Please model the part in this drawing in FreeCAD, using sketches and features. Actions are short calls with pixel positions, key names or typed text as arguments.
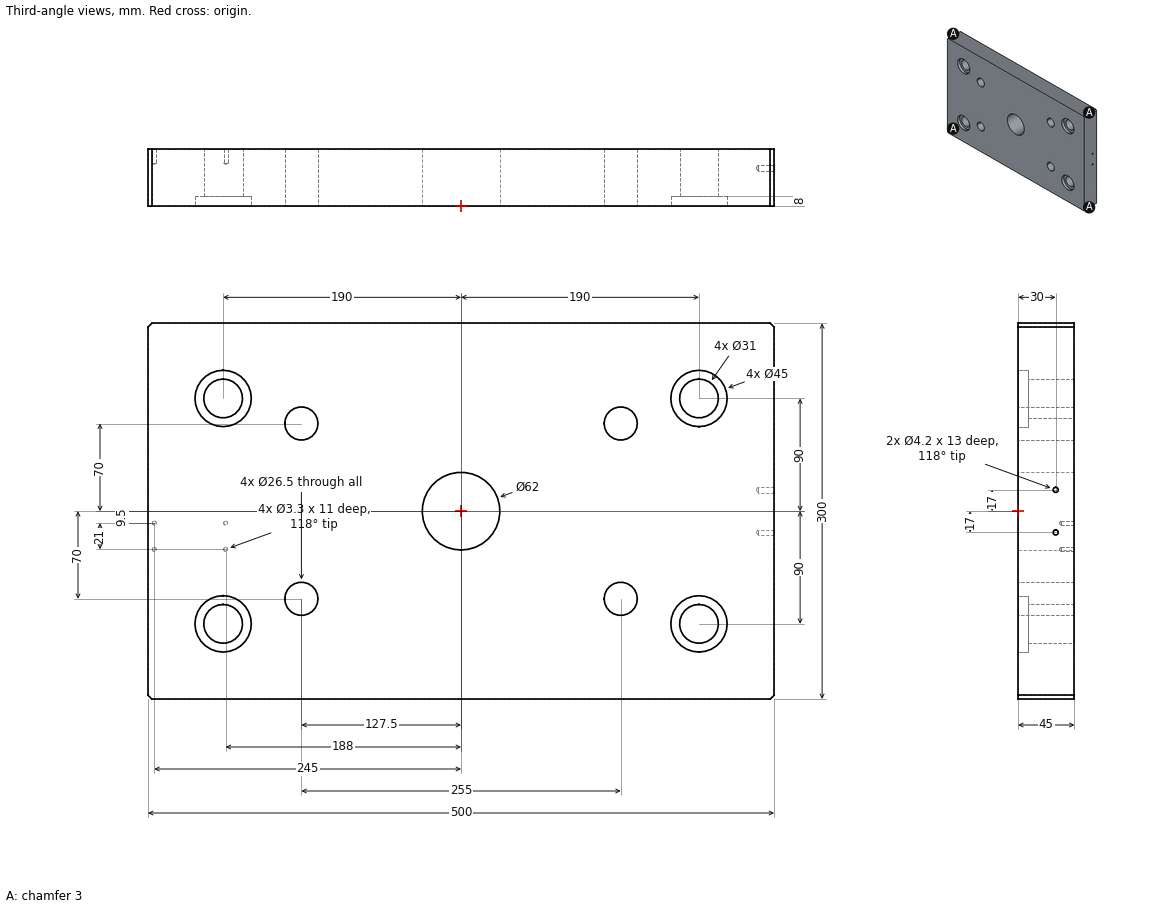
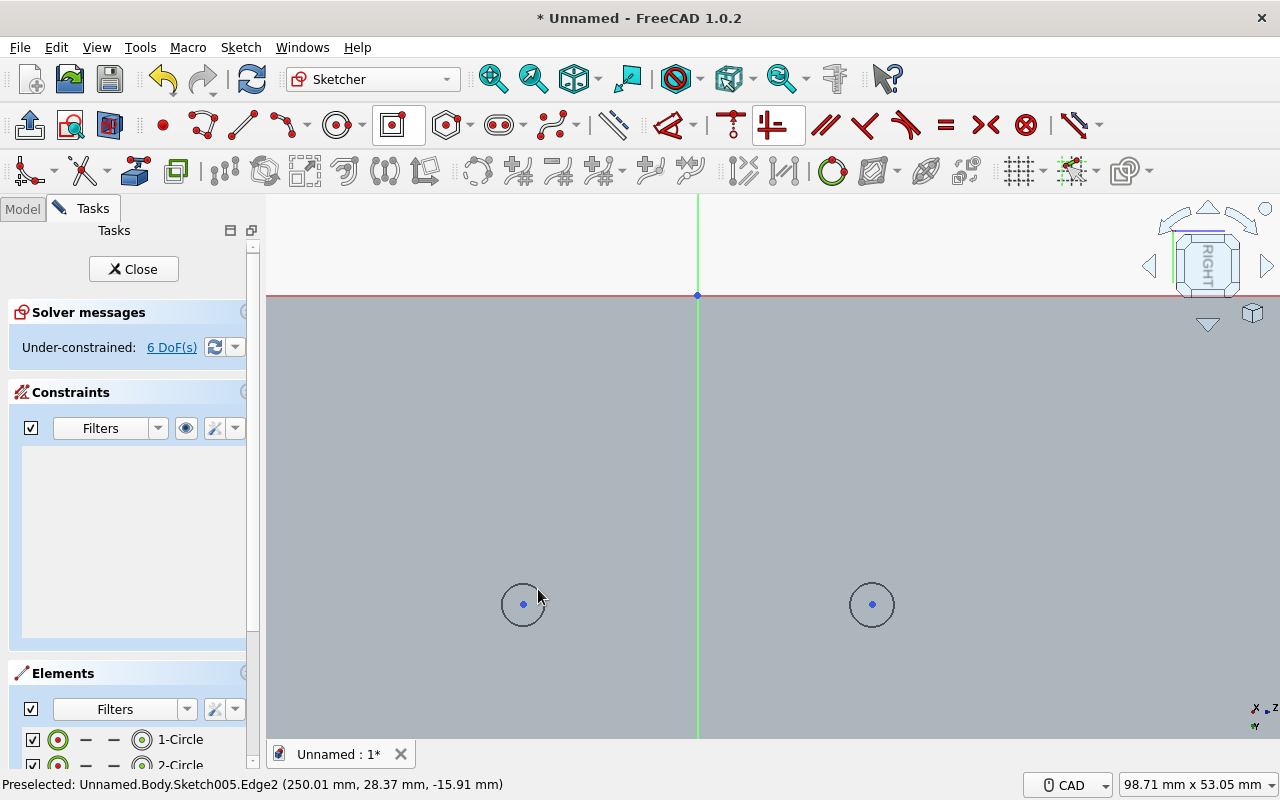
click(887, 589)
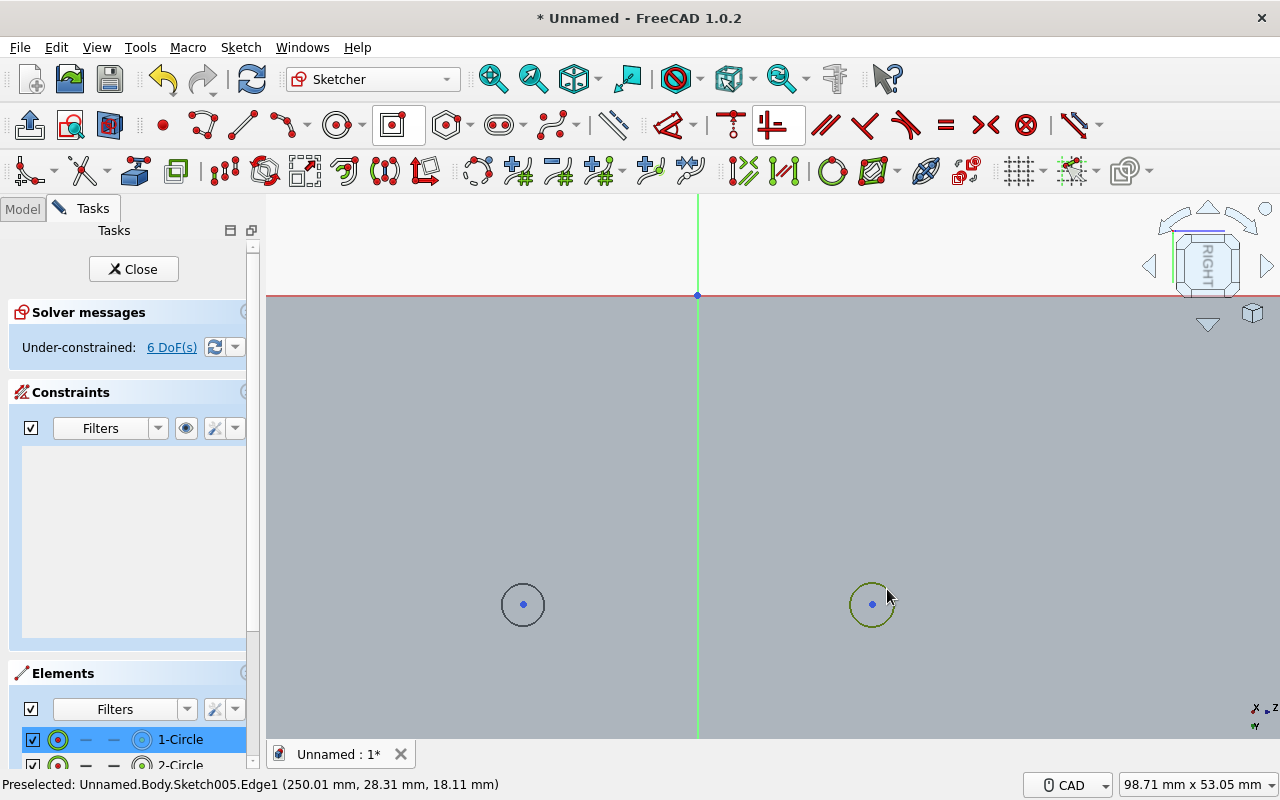
click(538, 590)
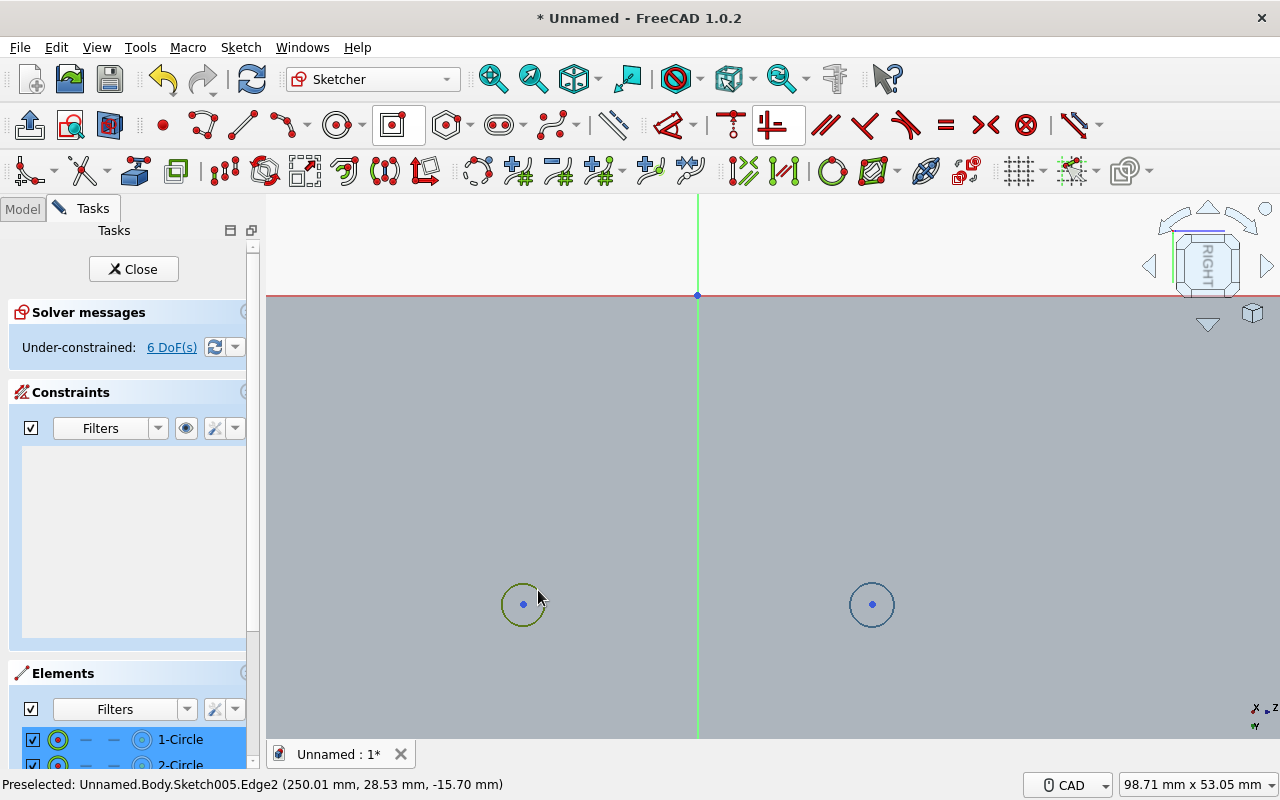
click(946, 126)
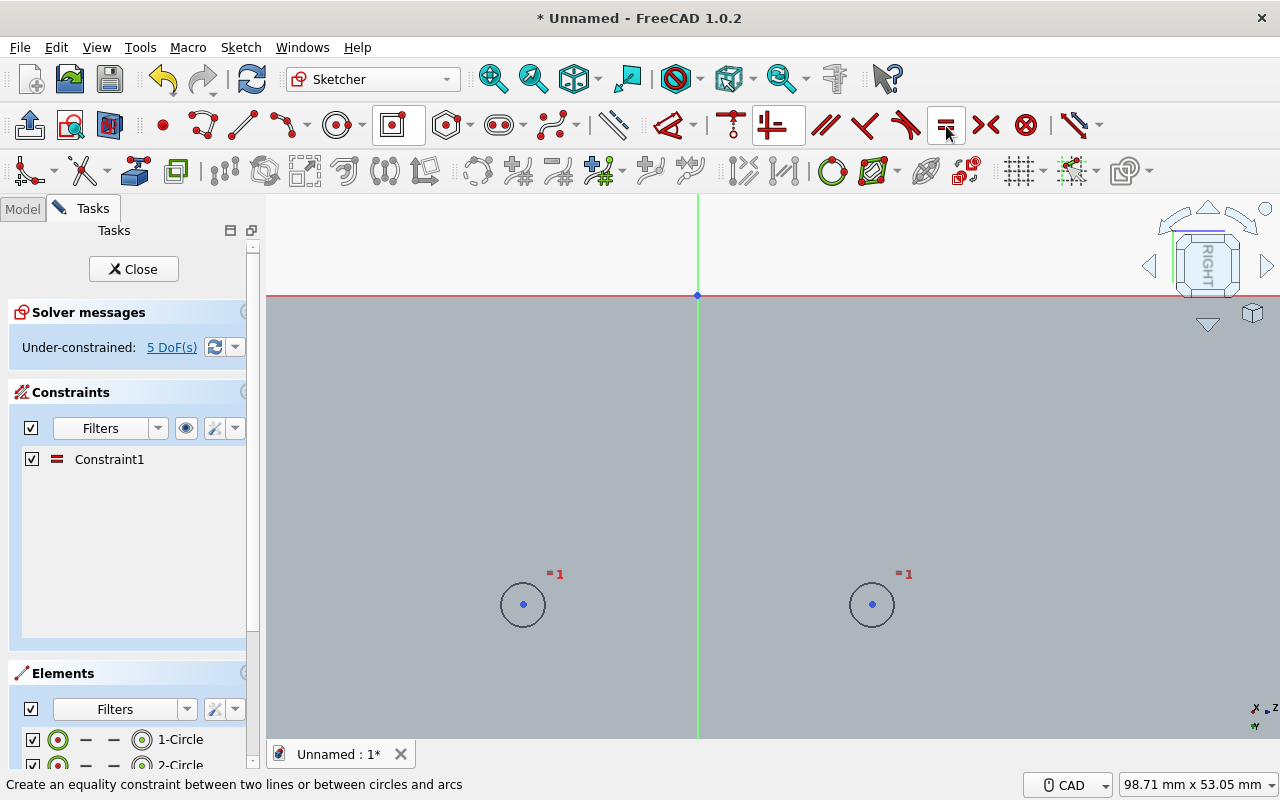
click(872, 605)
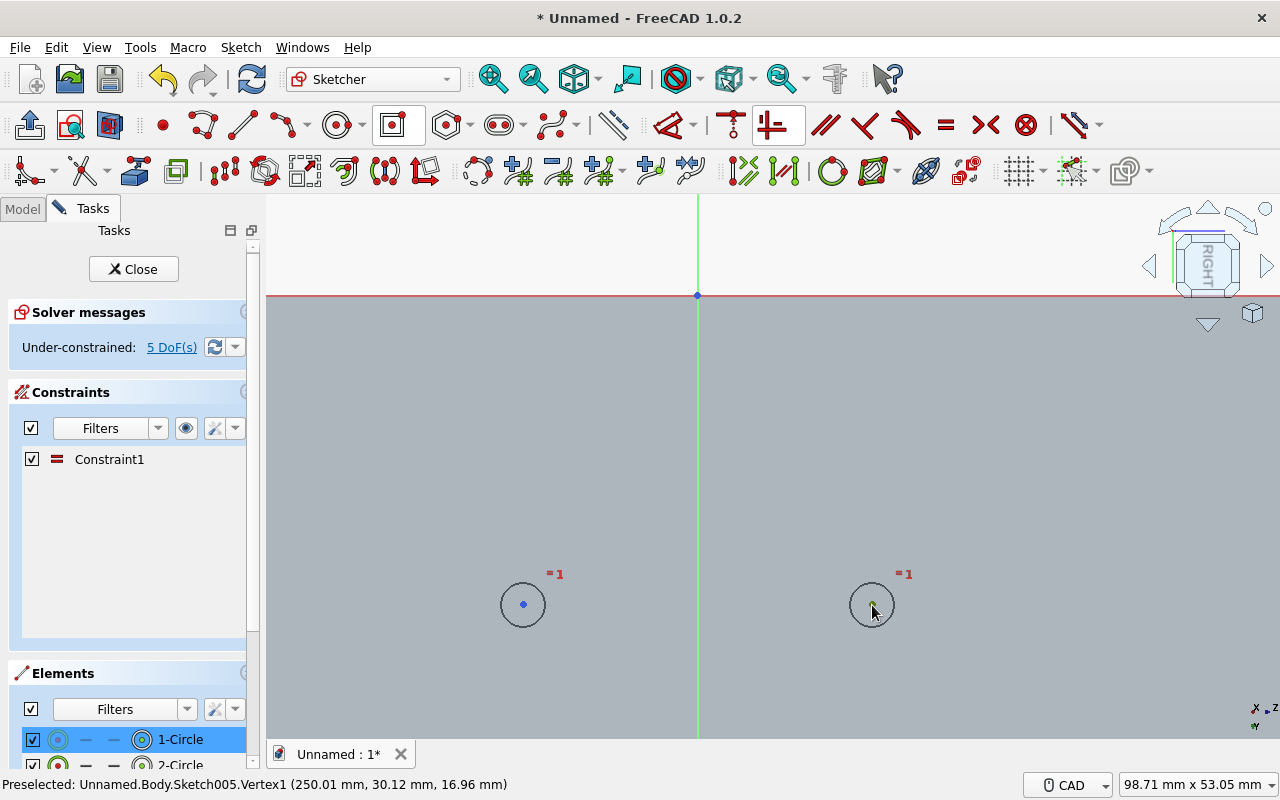
click(523, 605)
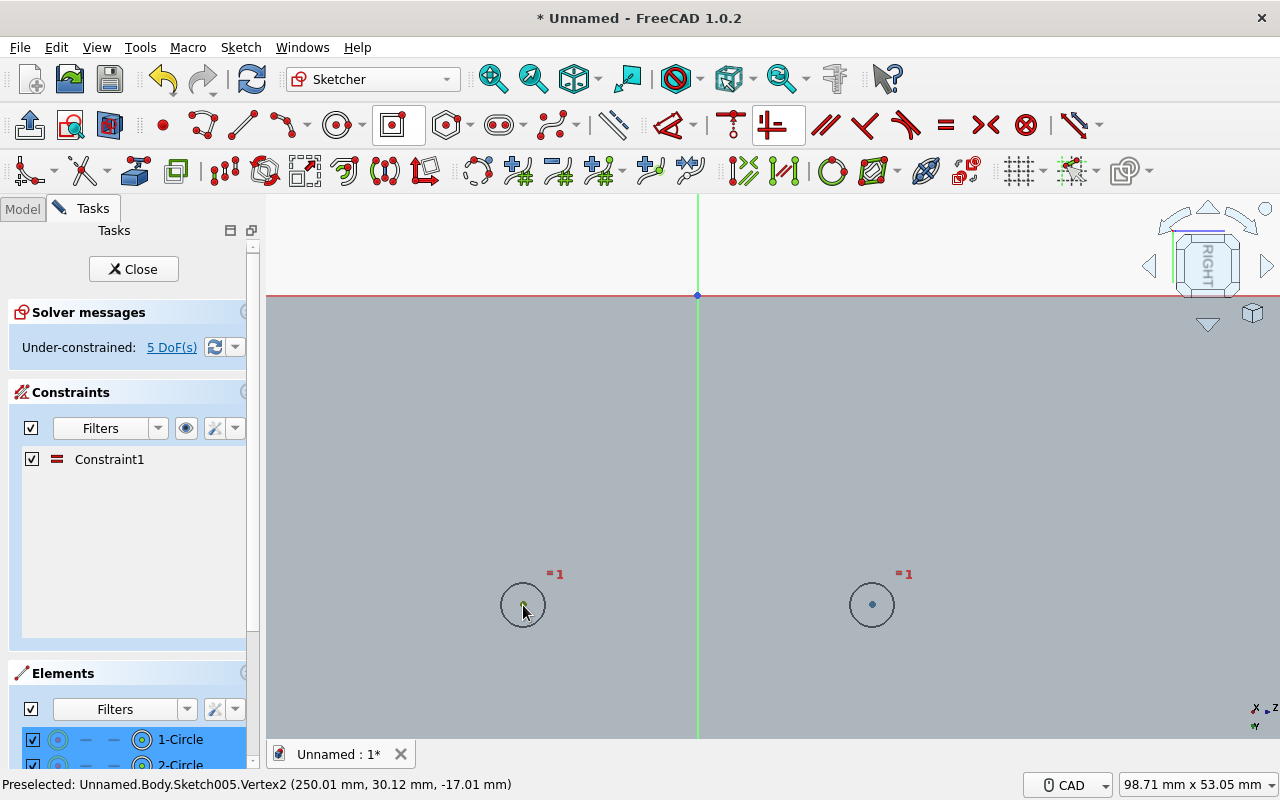
key(h)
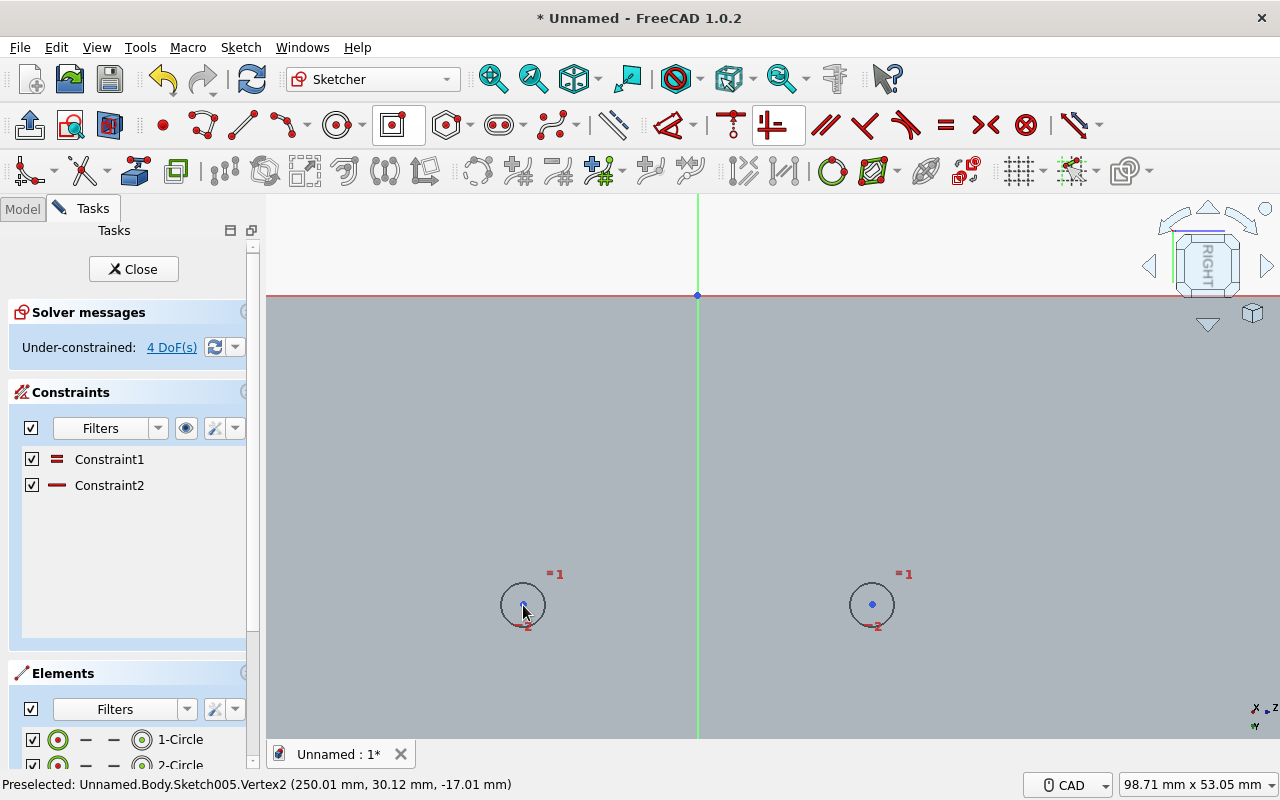
key(d)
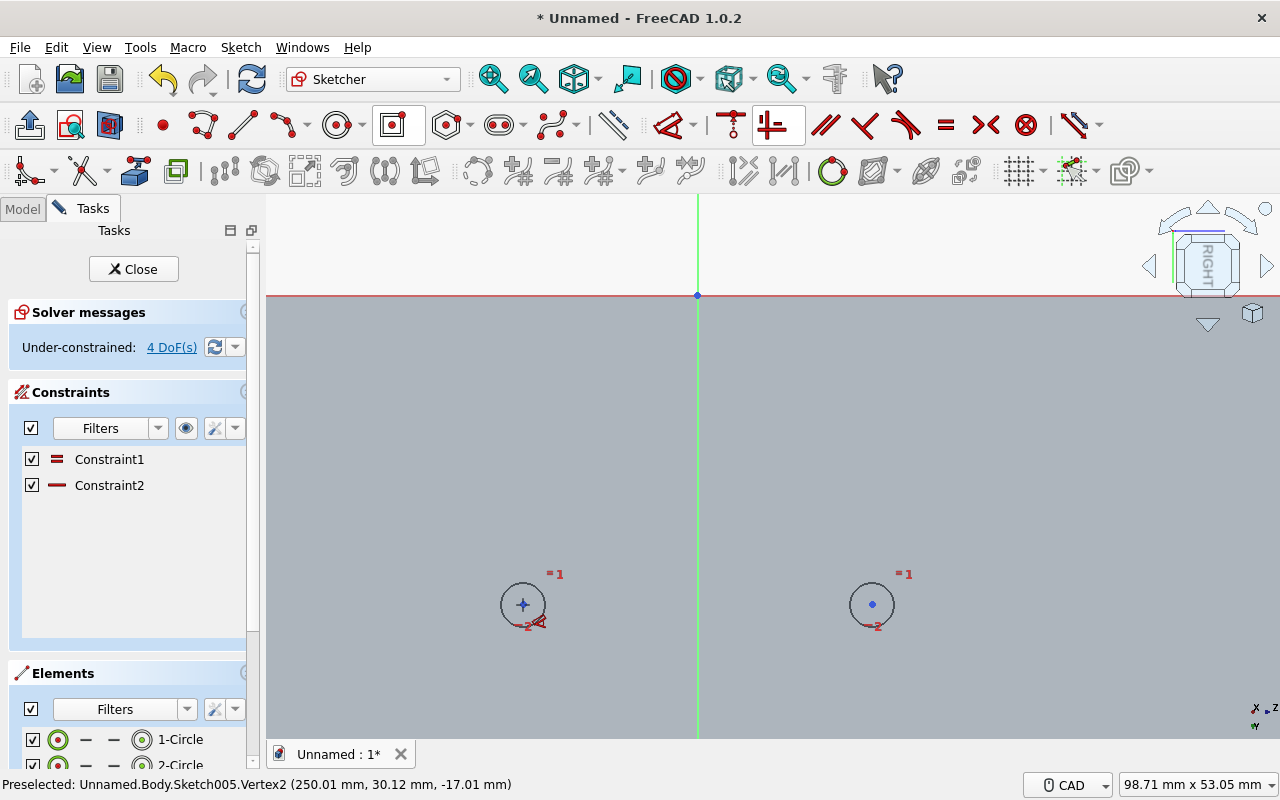
click(887, 589)
click(909, 566)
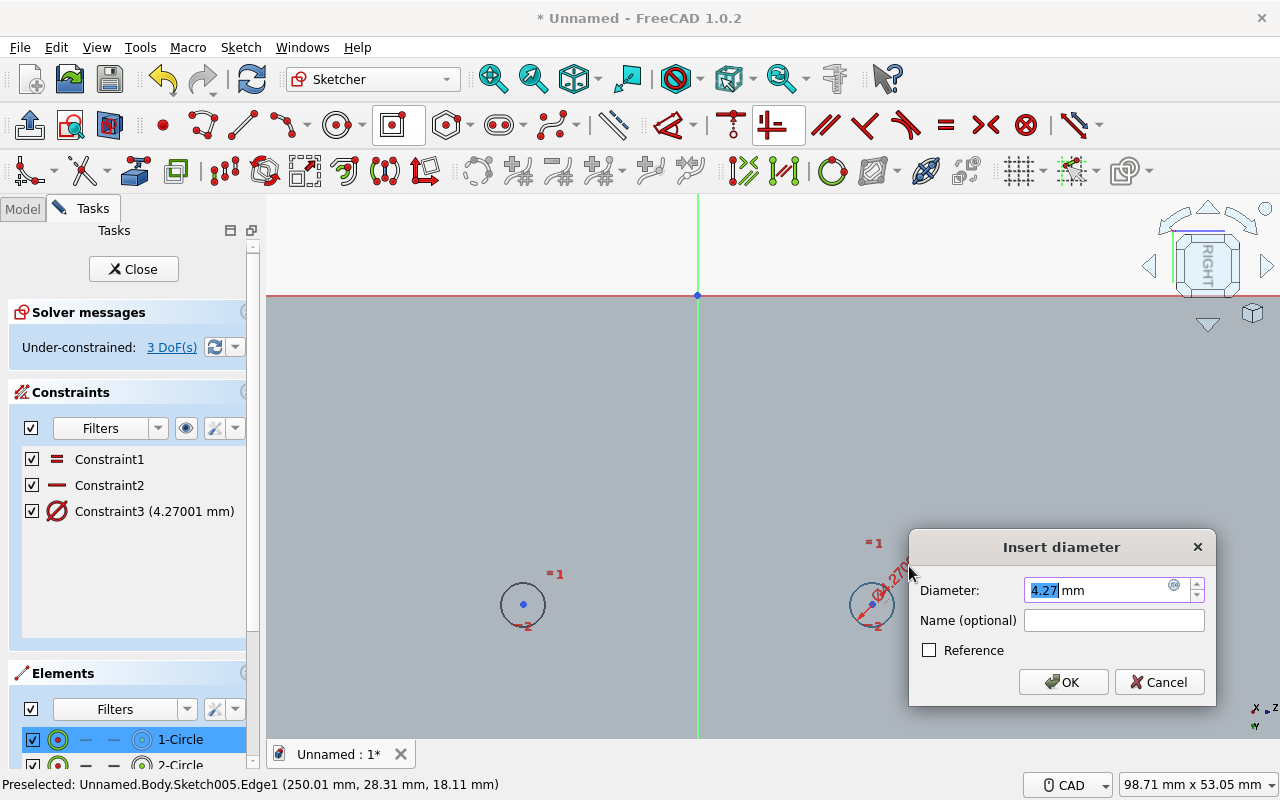
text(4.2)
key(Return)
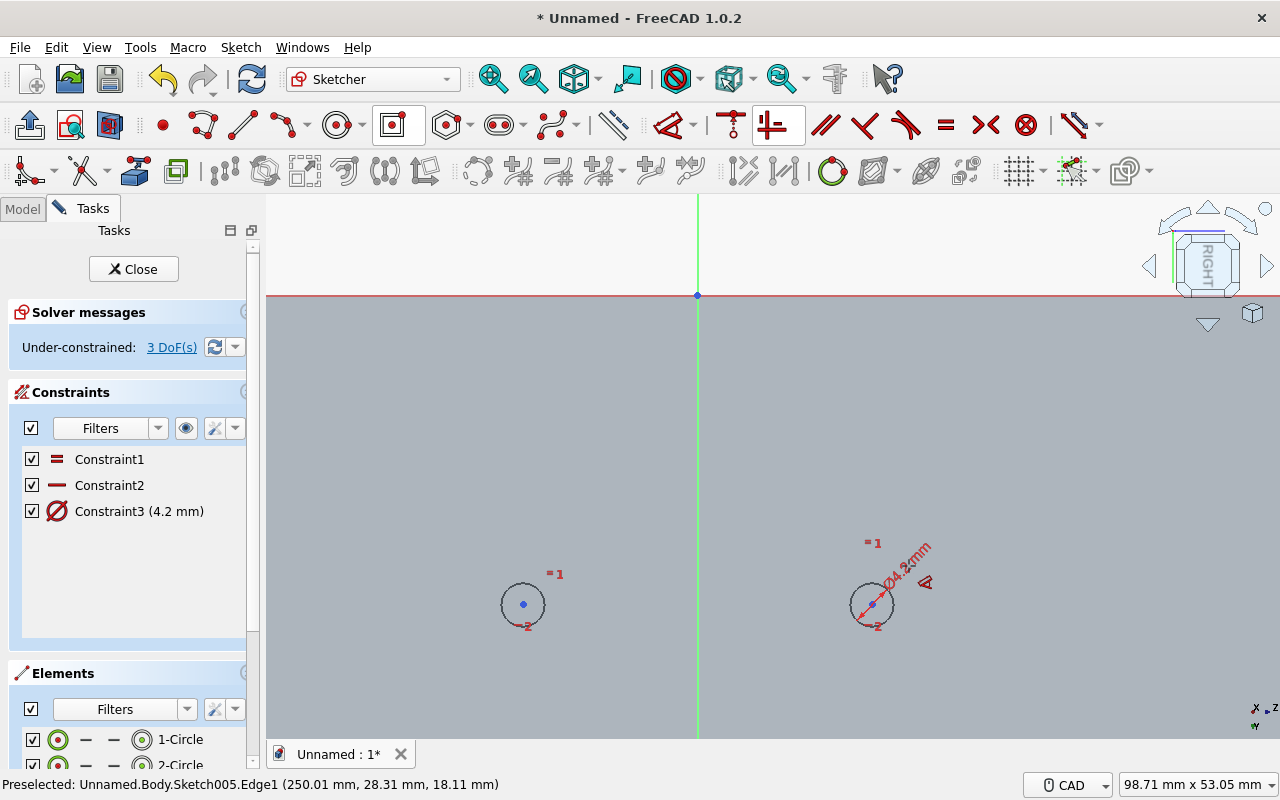
click(872, 605)
click(785, 262)